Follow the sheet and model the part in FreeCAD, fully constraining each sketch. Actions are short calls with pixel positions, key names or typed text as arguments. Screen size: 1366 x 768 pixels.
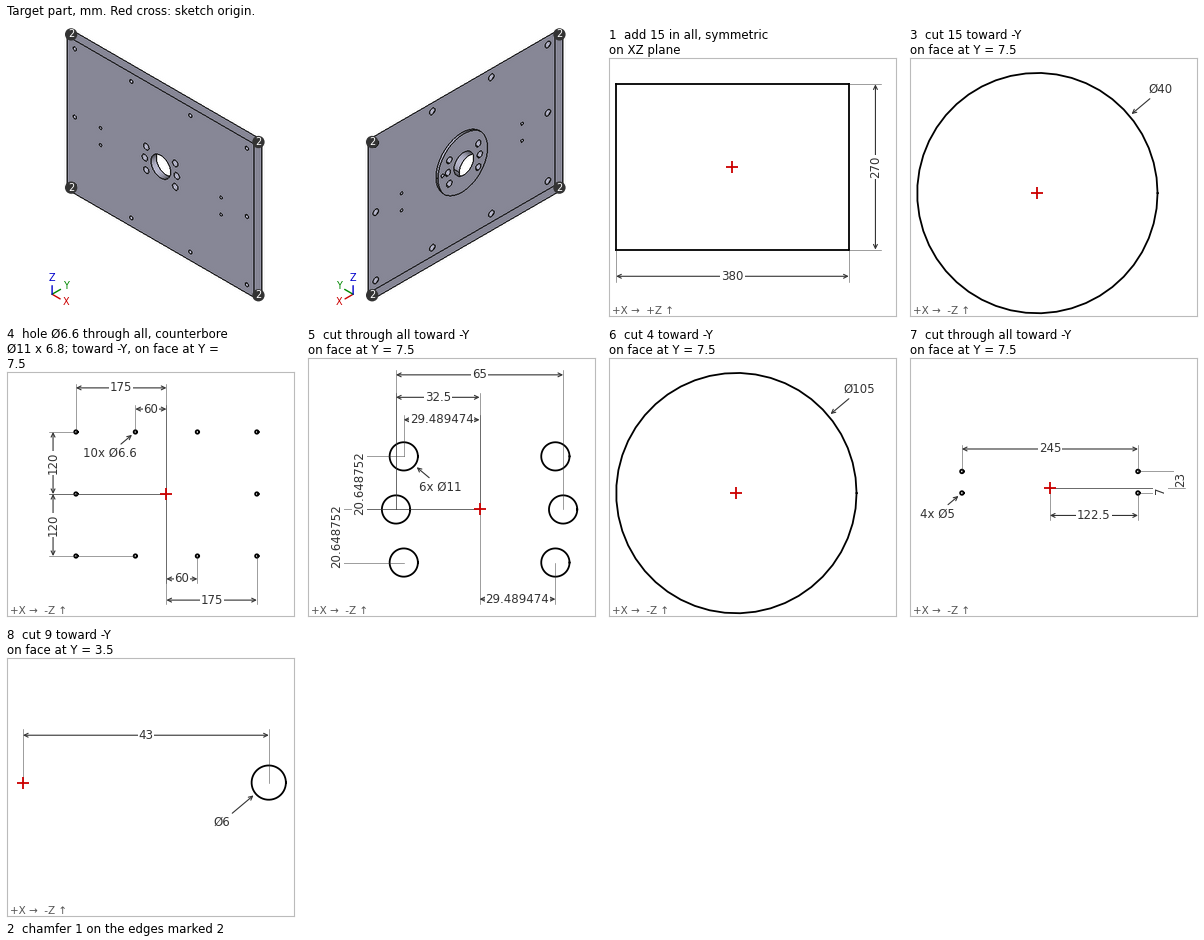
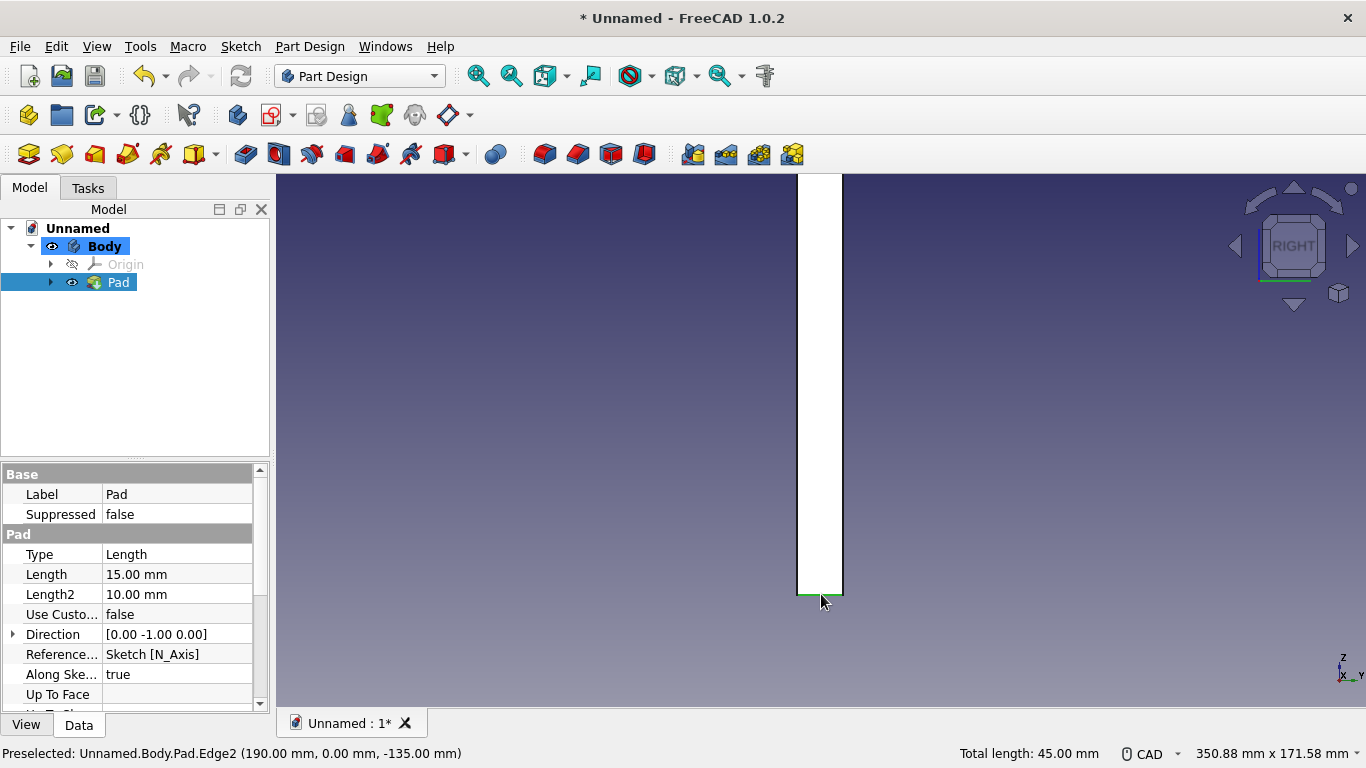
click(479, 76)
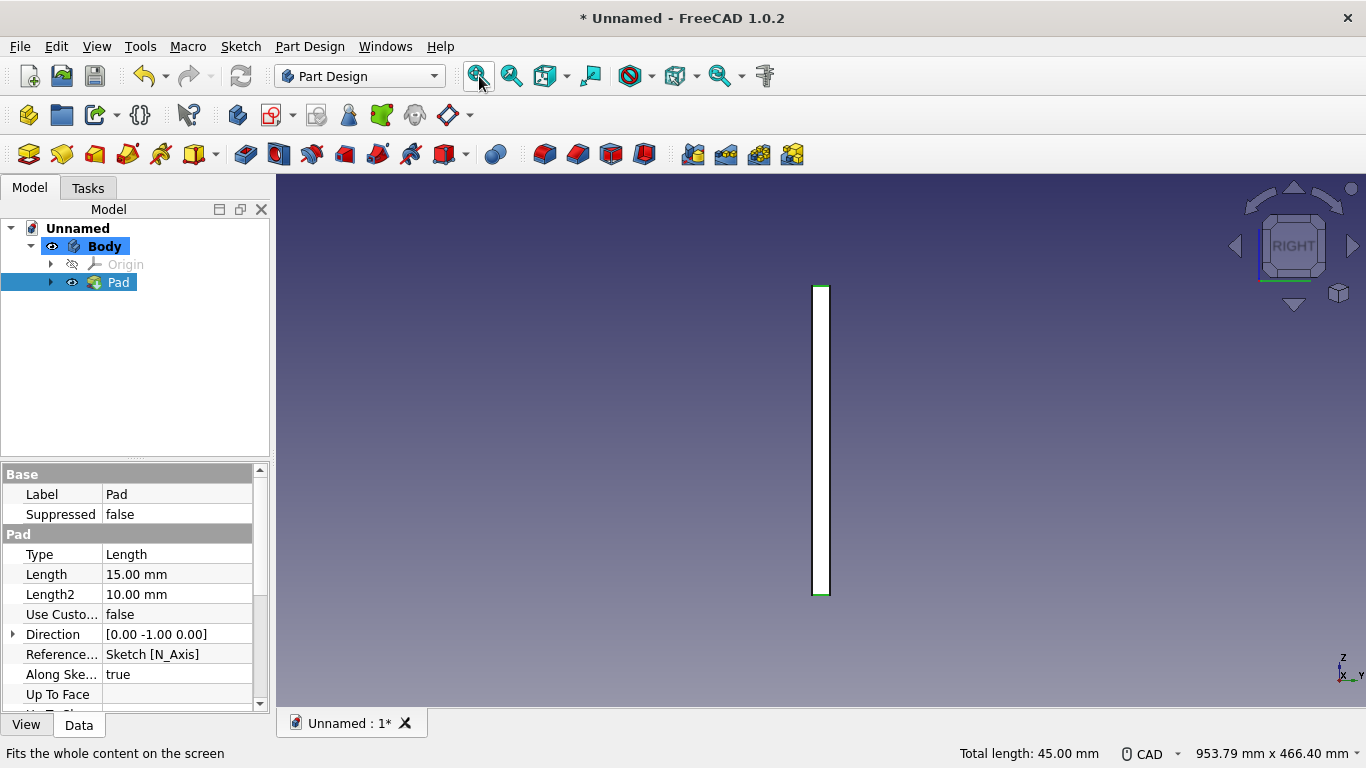
key(5)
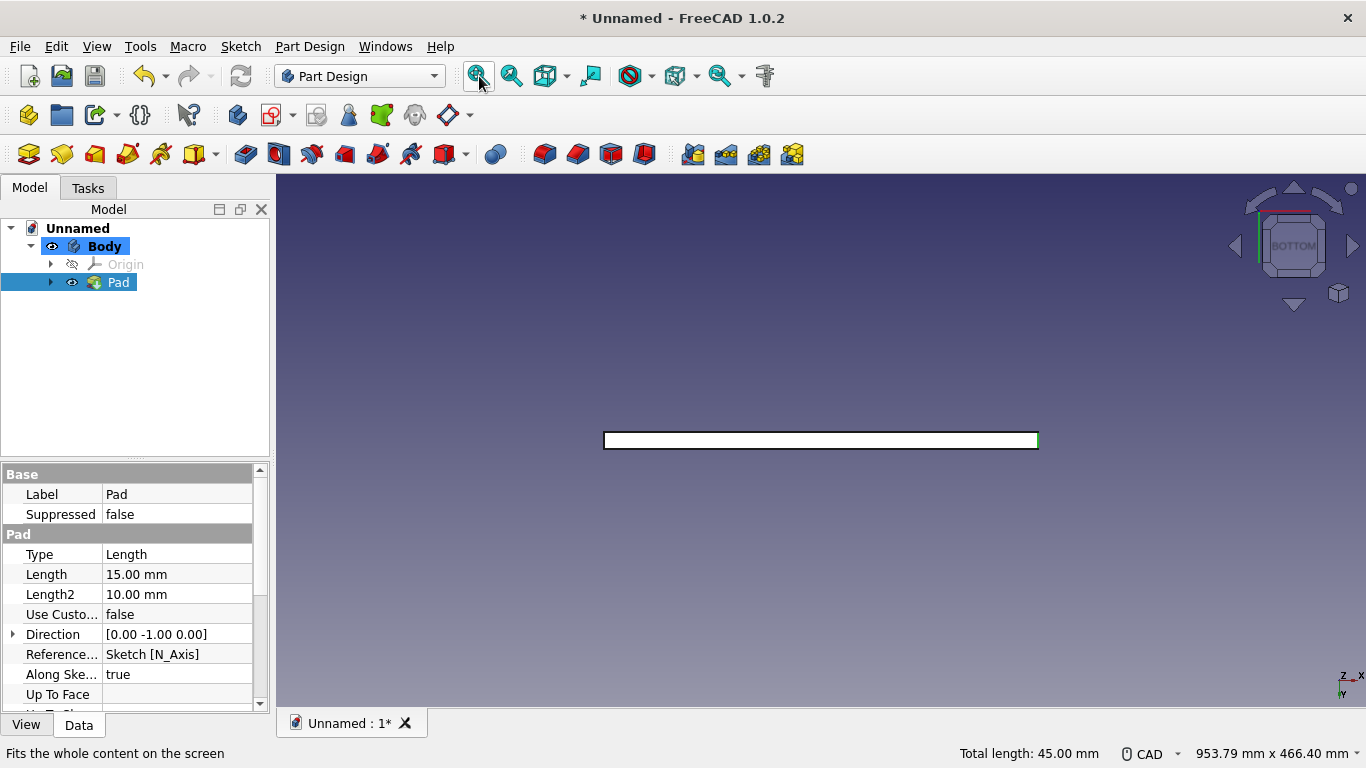
click(479, 76)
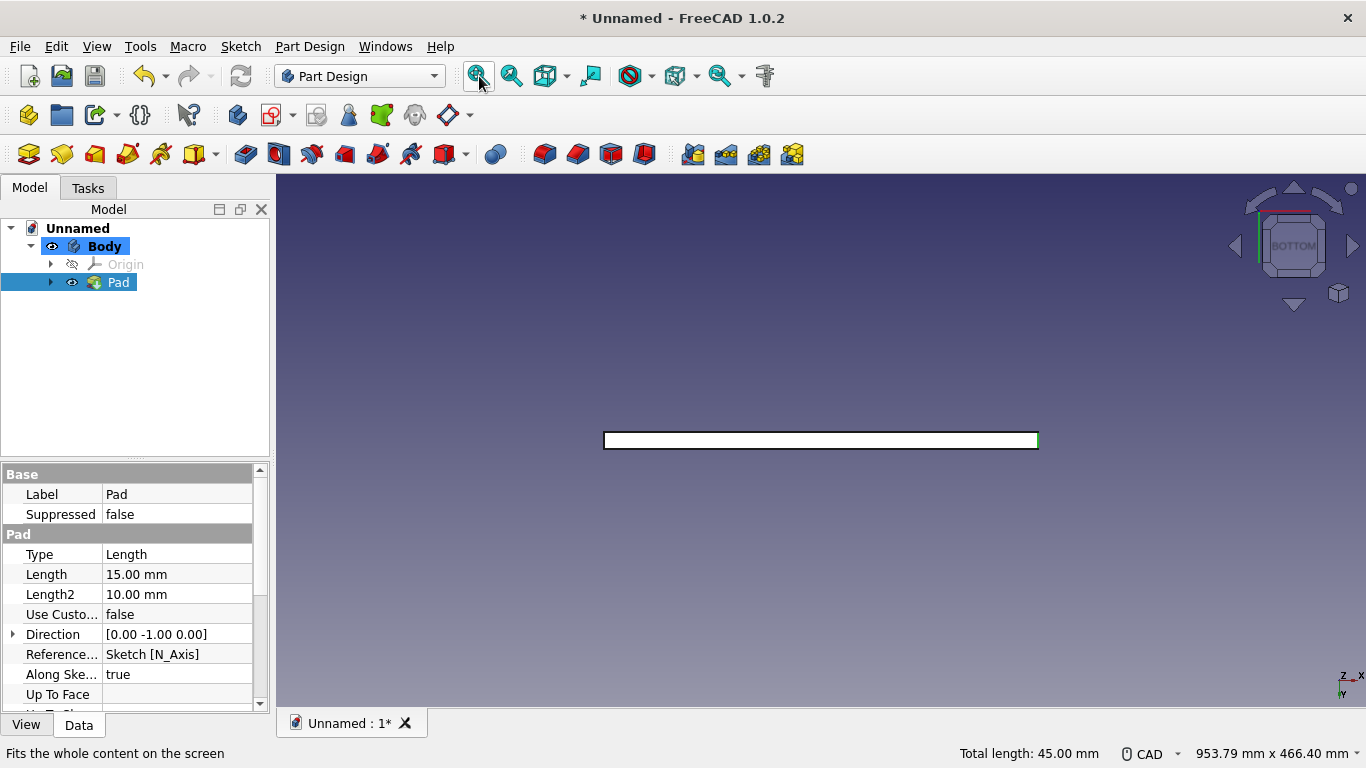
click(604, 439, ctrl)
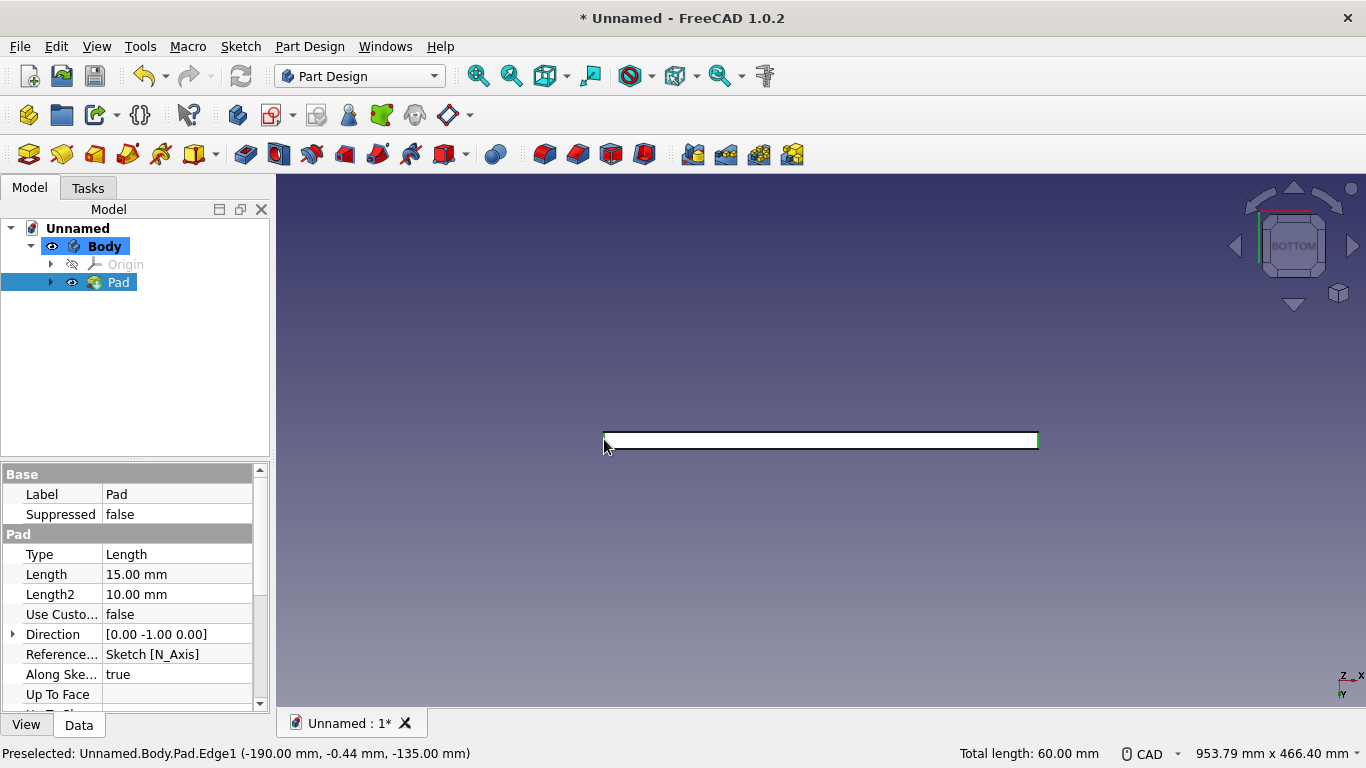
click(578, 154)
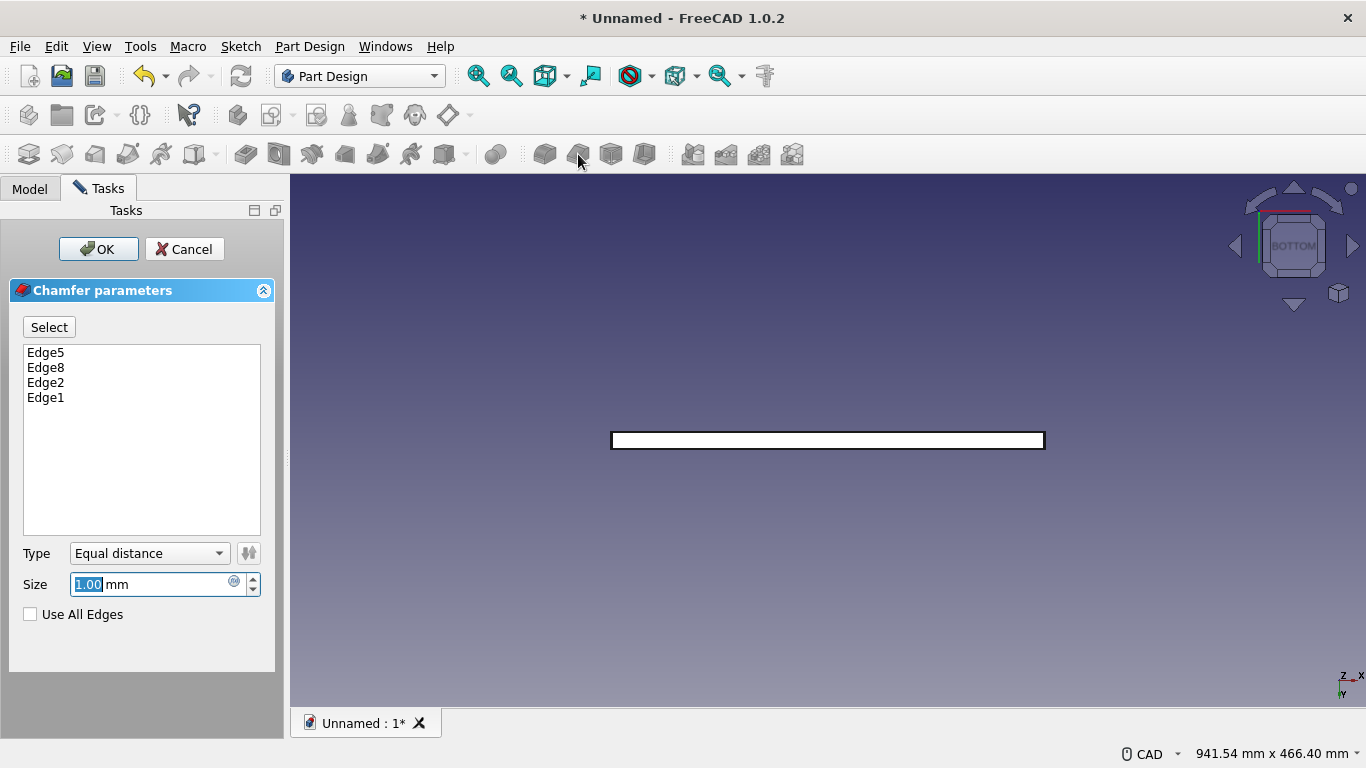
text(1)
key(Tab)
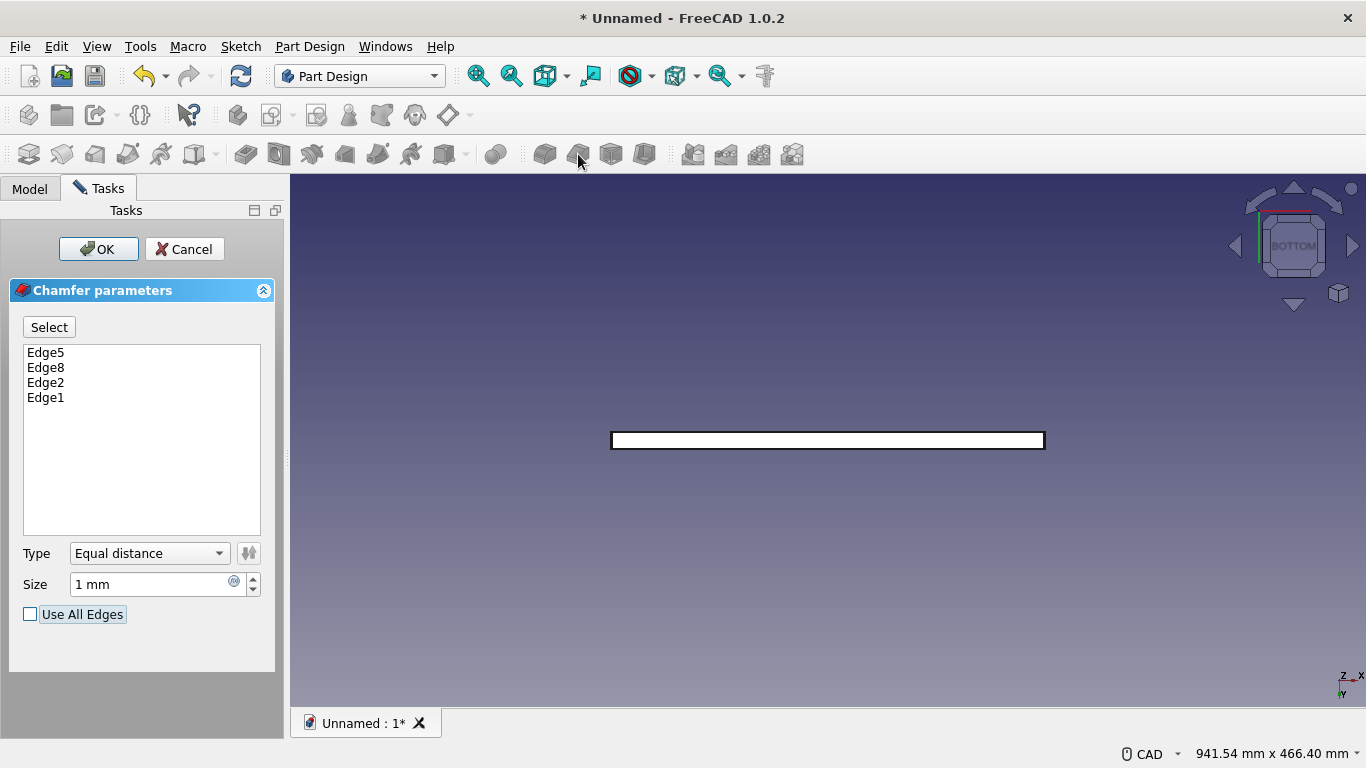
click(99, 249)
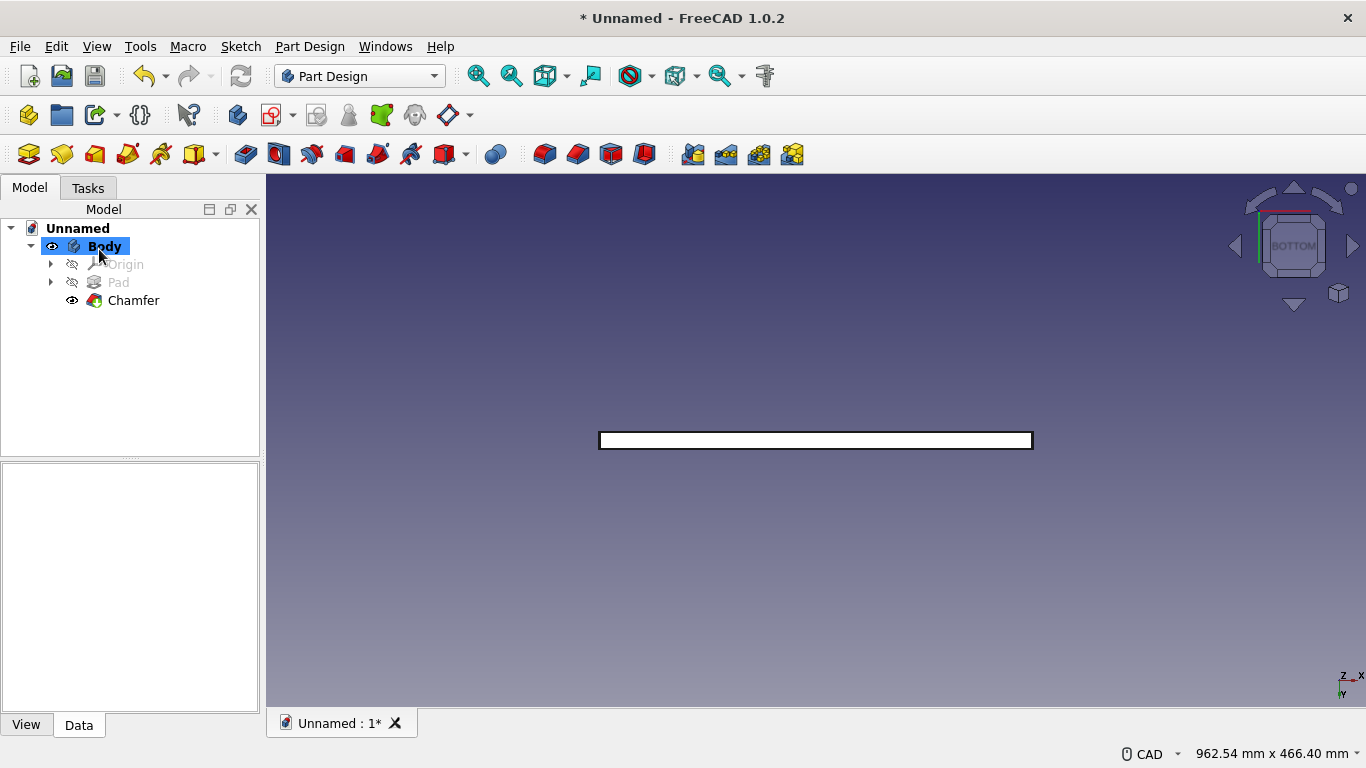
click(479, 76)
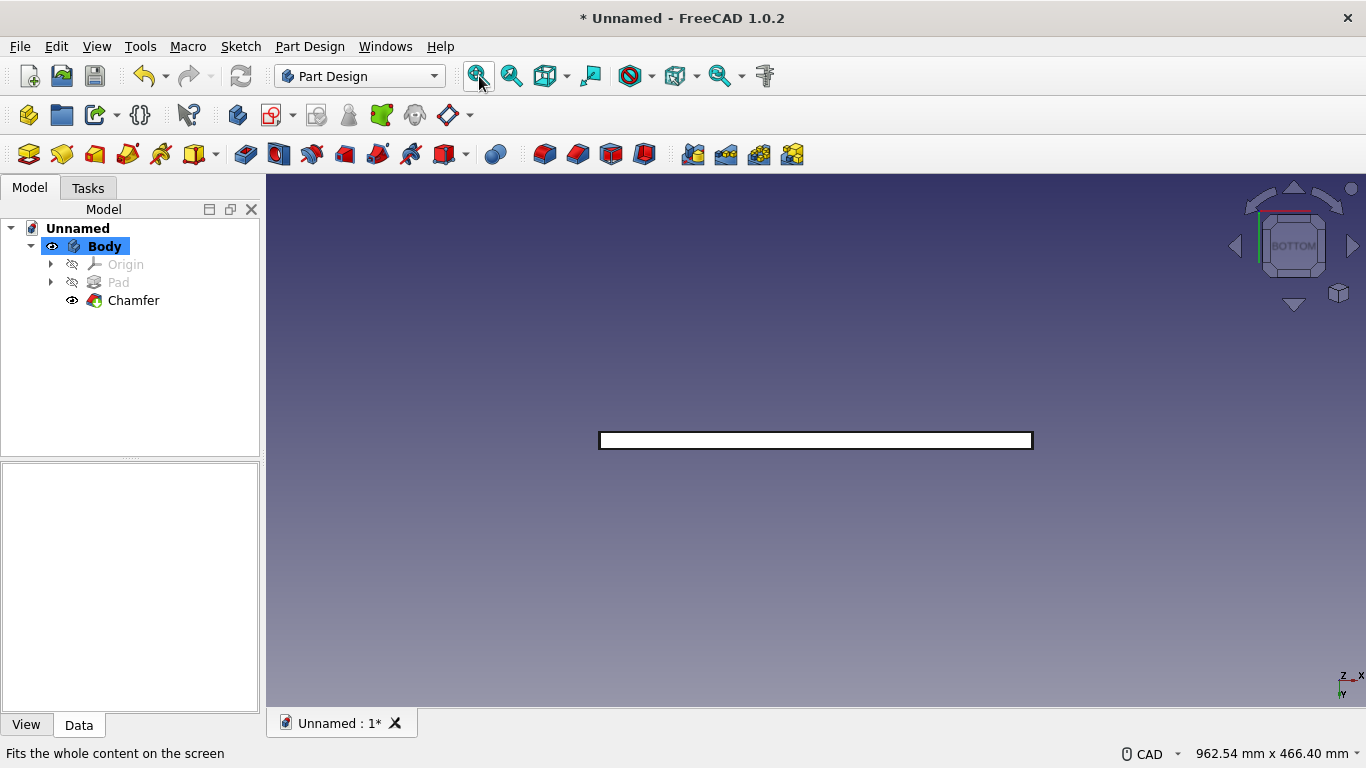
key(4)